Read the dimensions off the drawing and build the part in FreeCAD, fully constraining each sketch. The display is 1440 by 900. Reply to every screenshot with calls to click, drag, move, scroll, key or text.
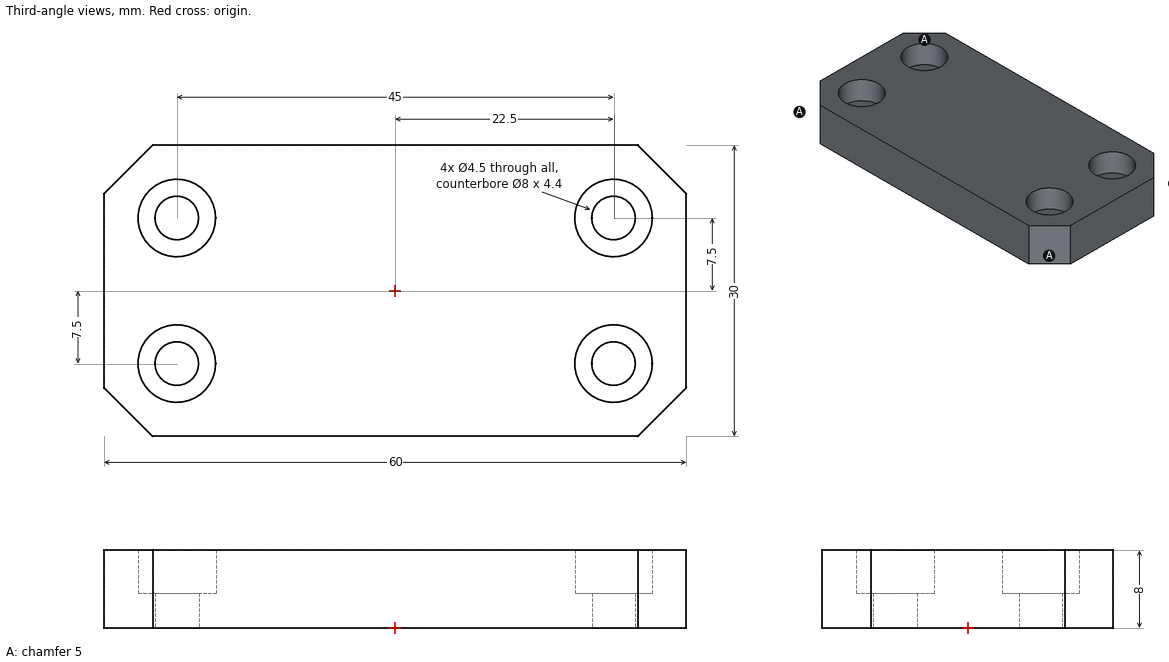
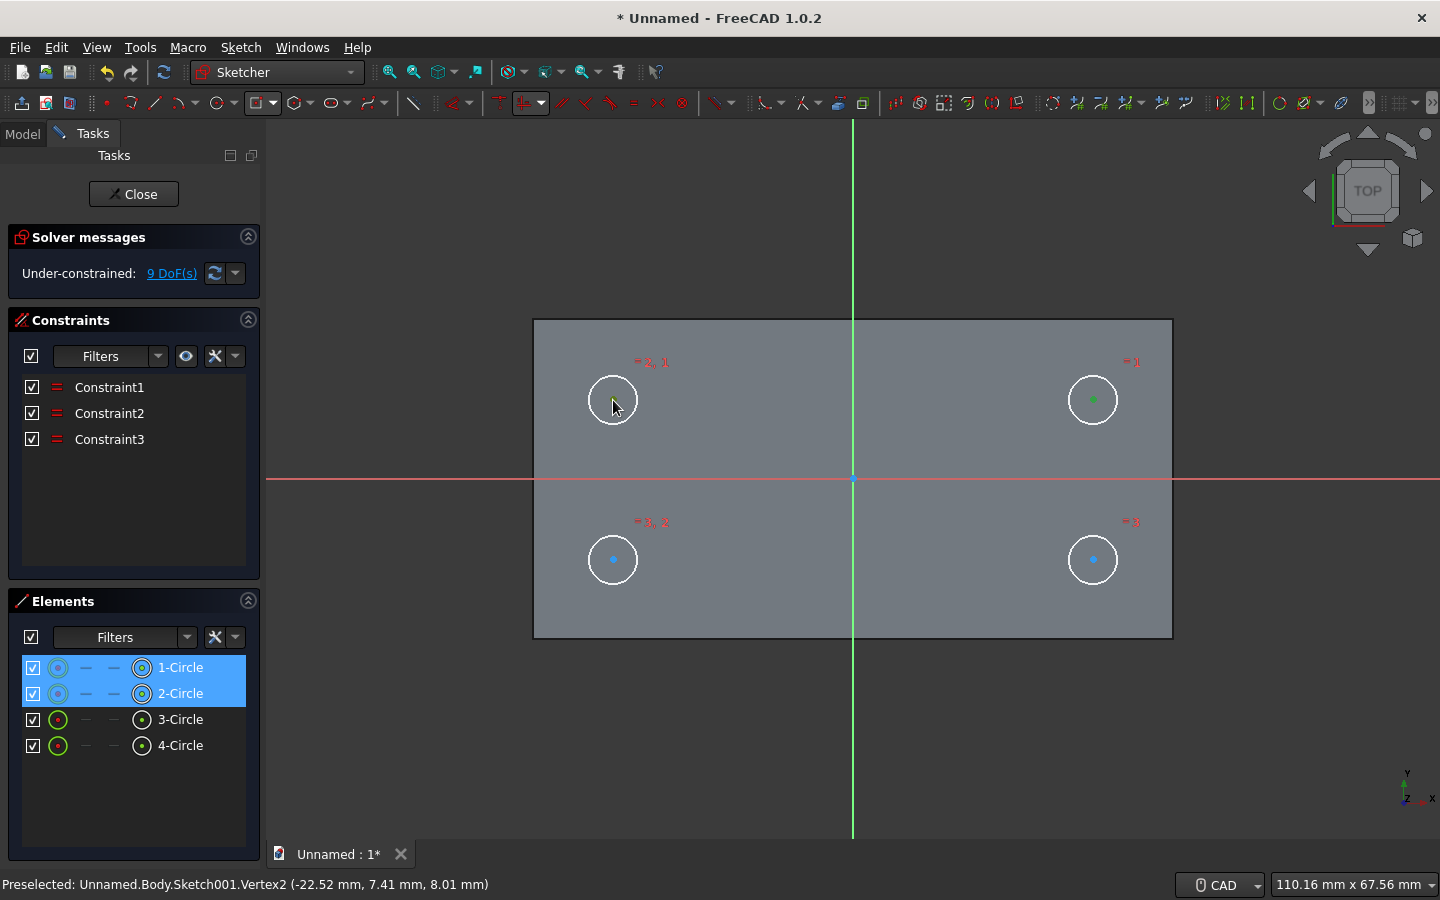
click(544, 104)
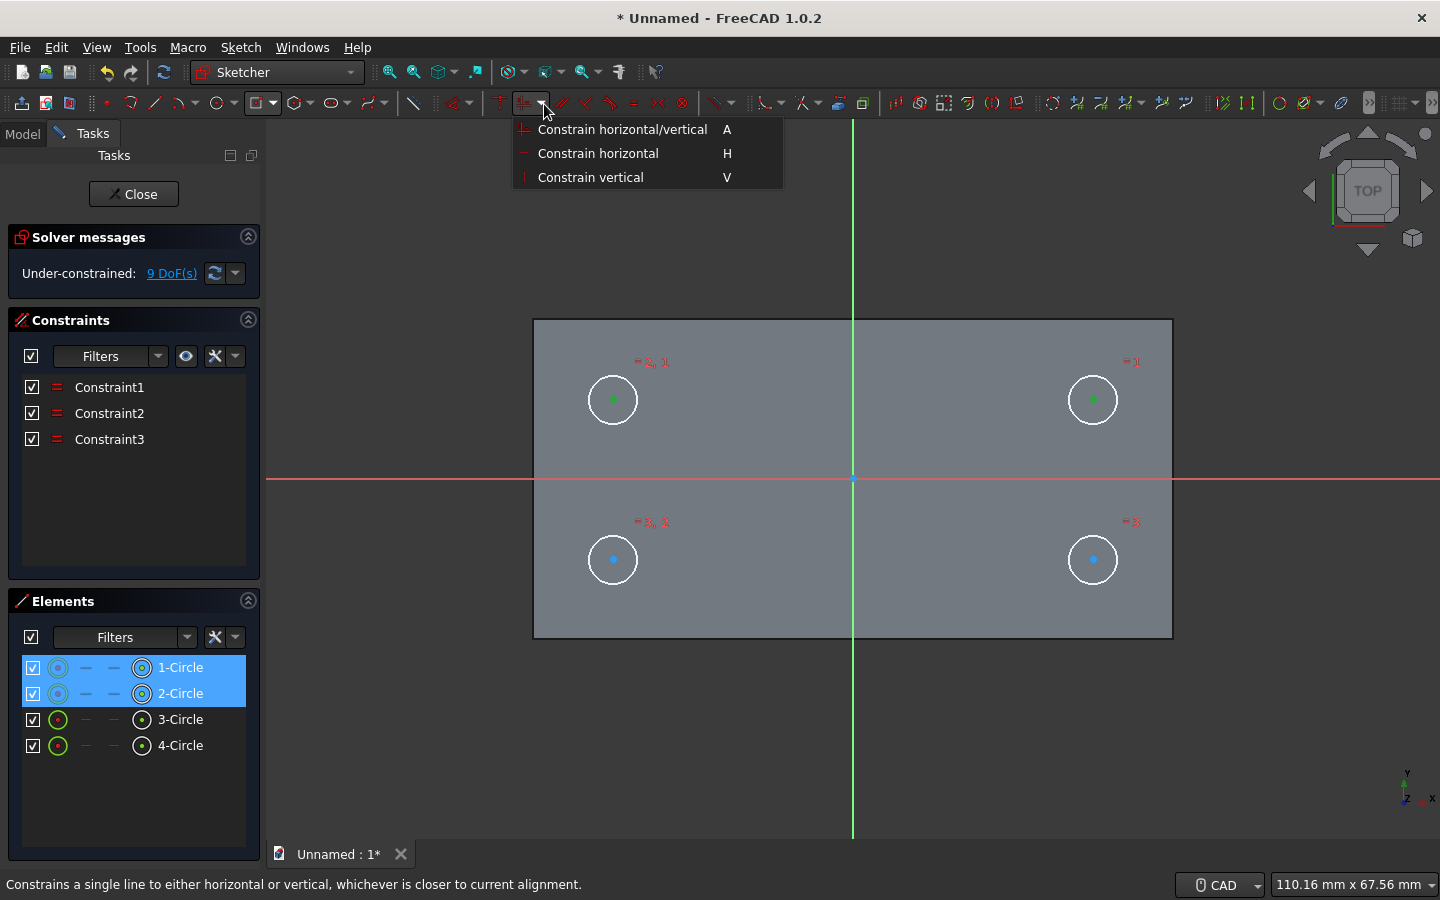
click(648, 153)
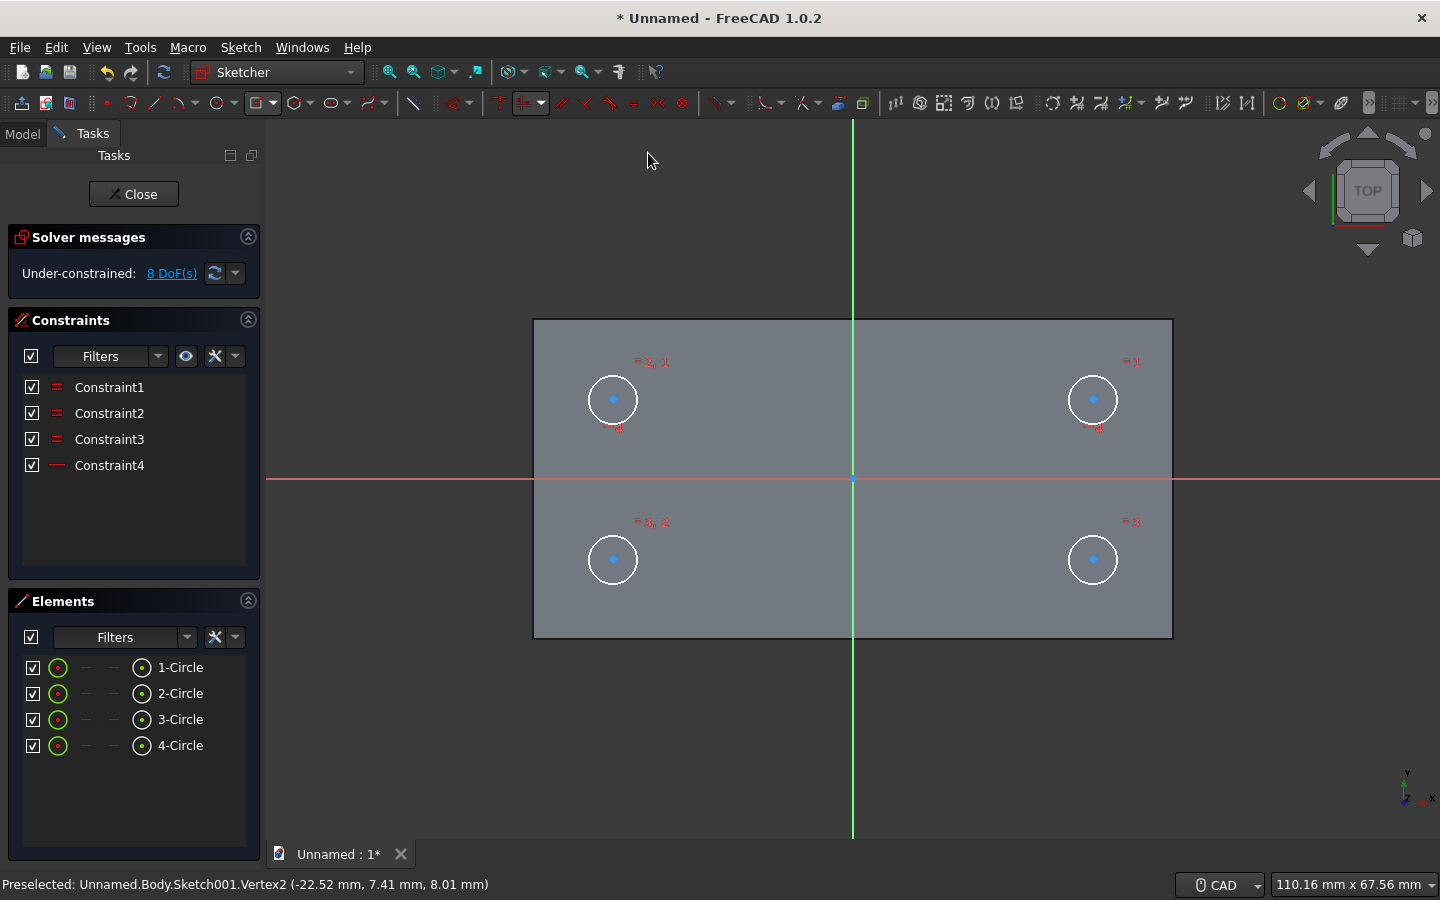
click(613, 400)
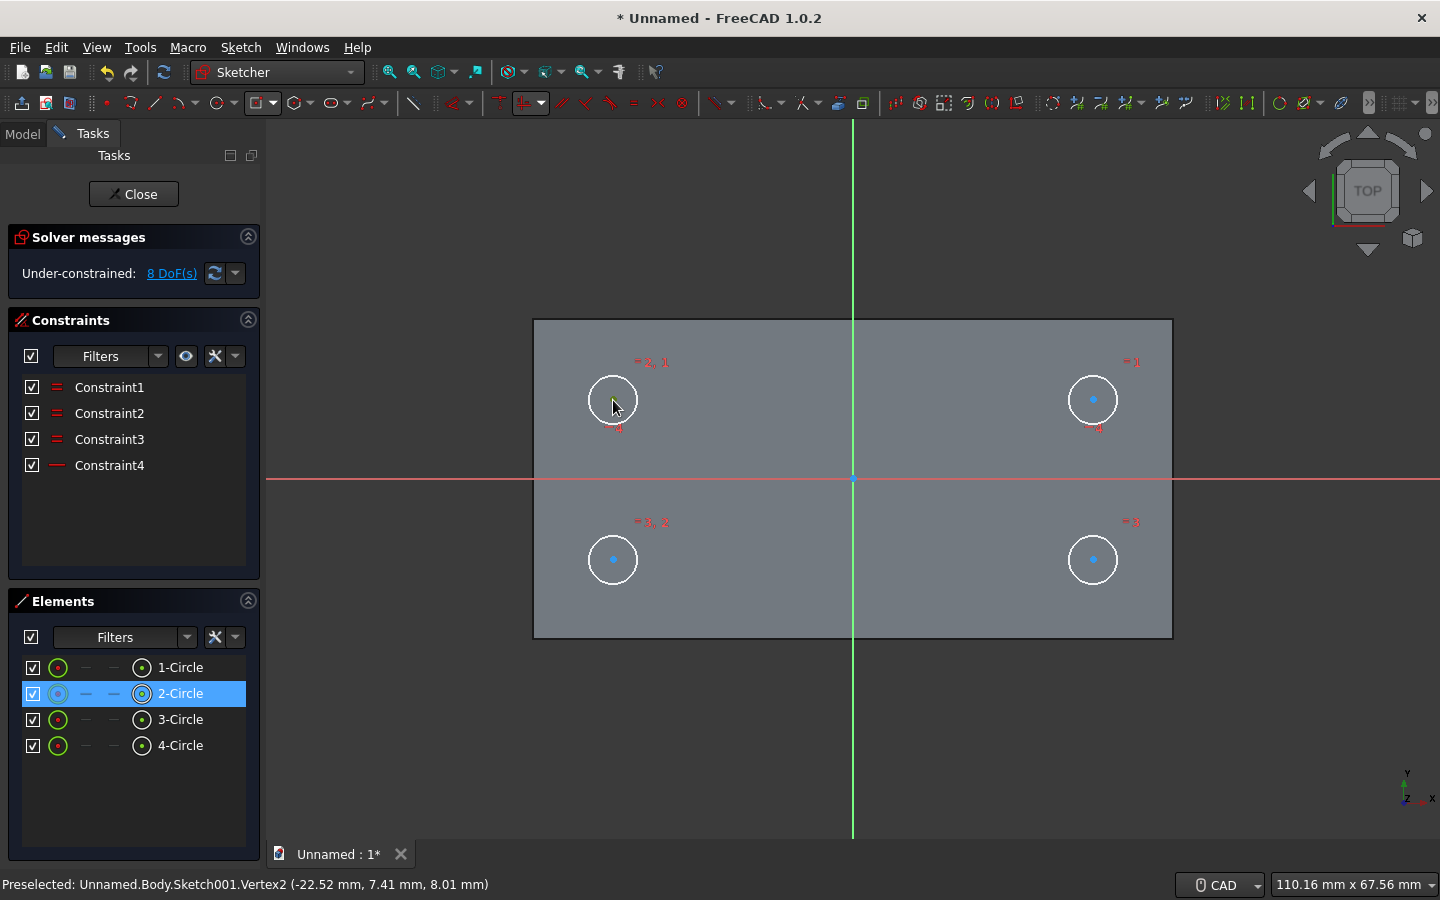
click(613, 560)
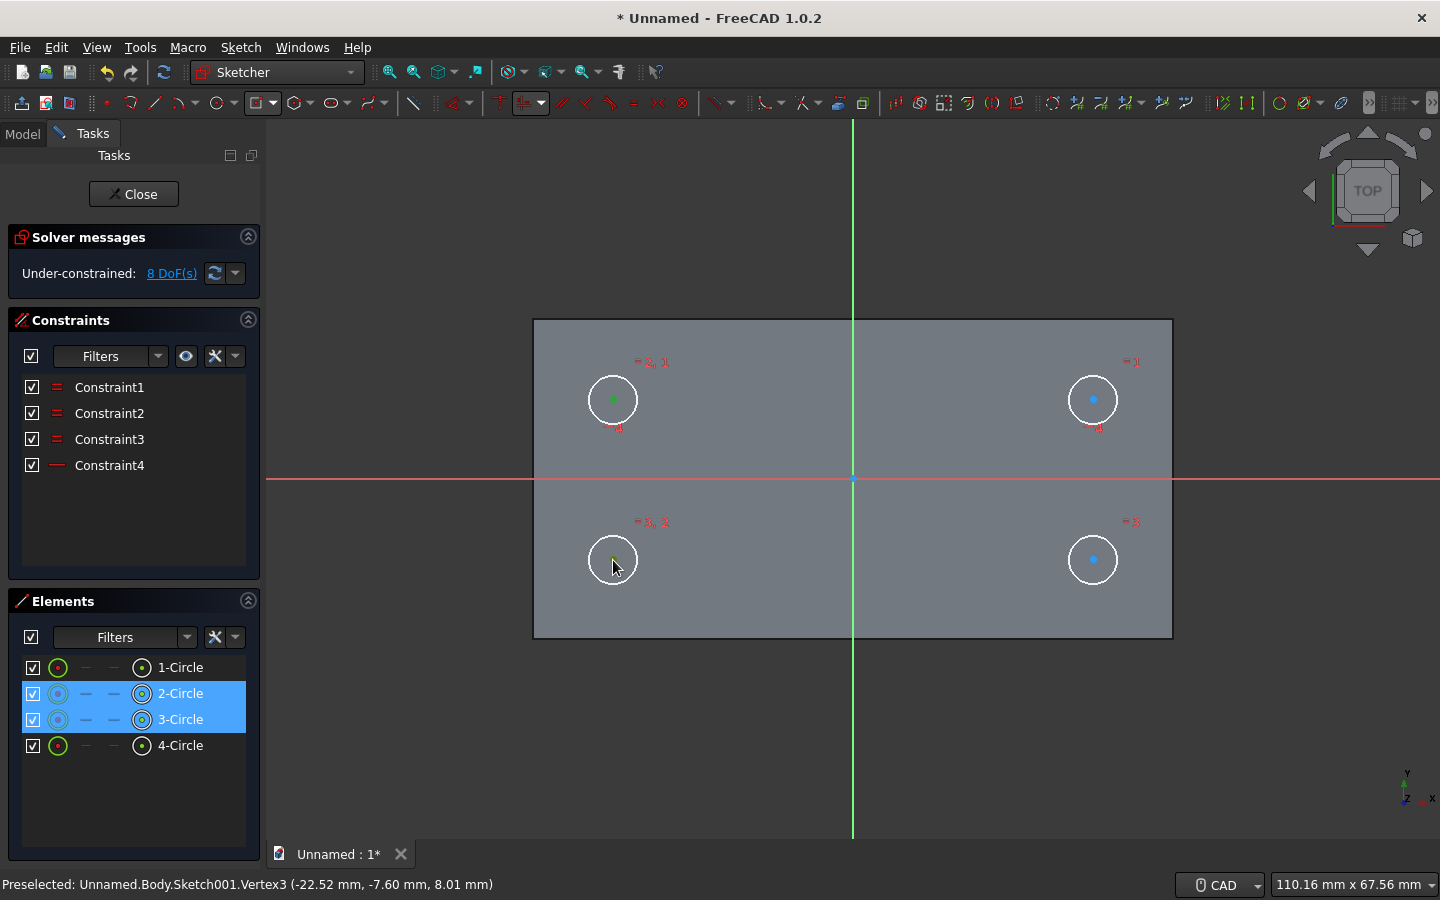
key(v)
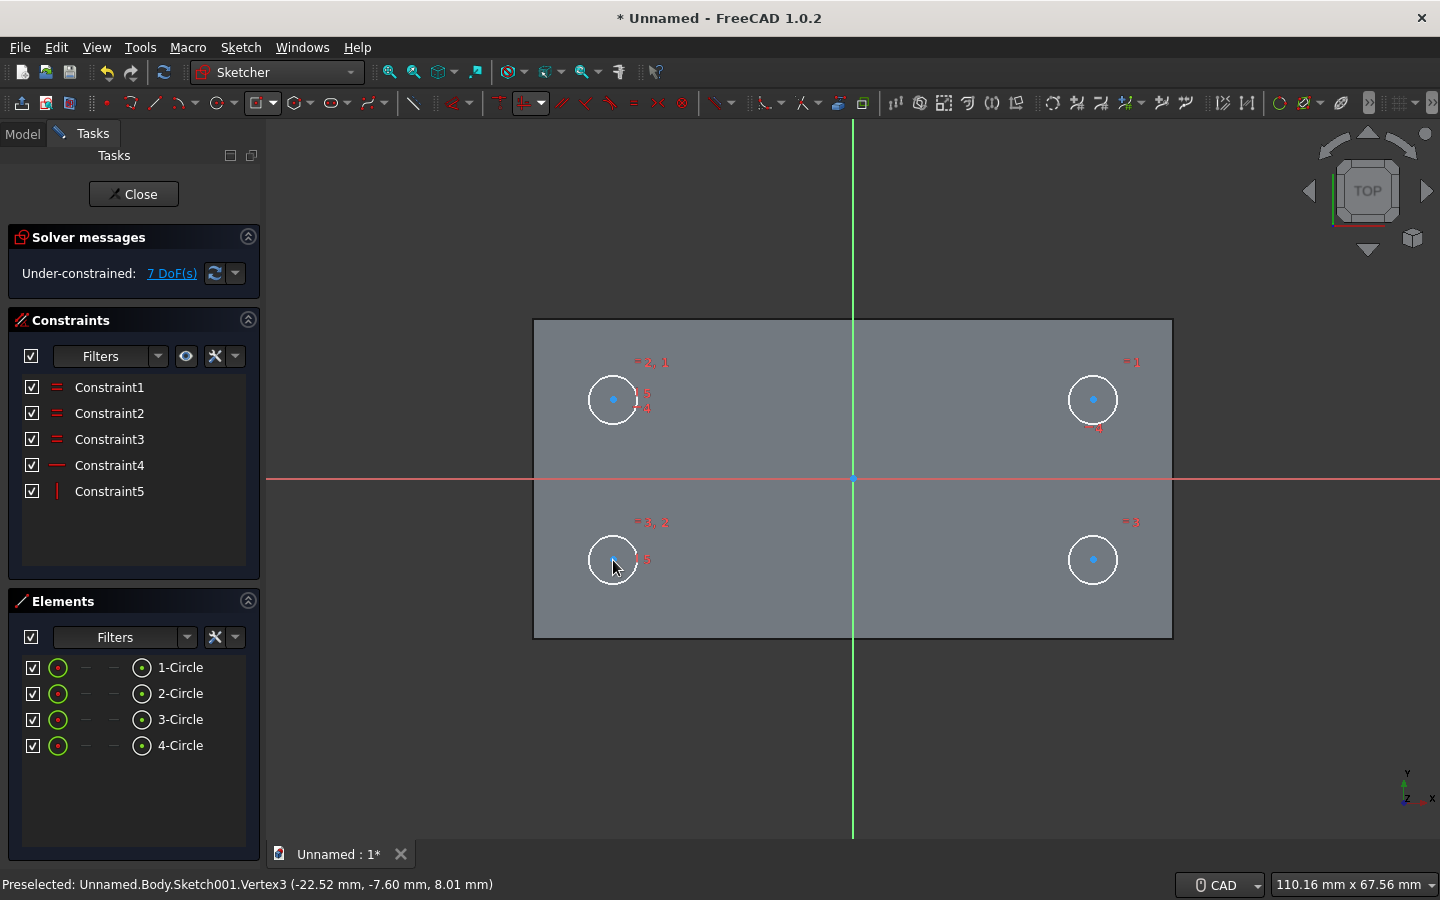
click(1093, 400)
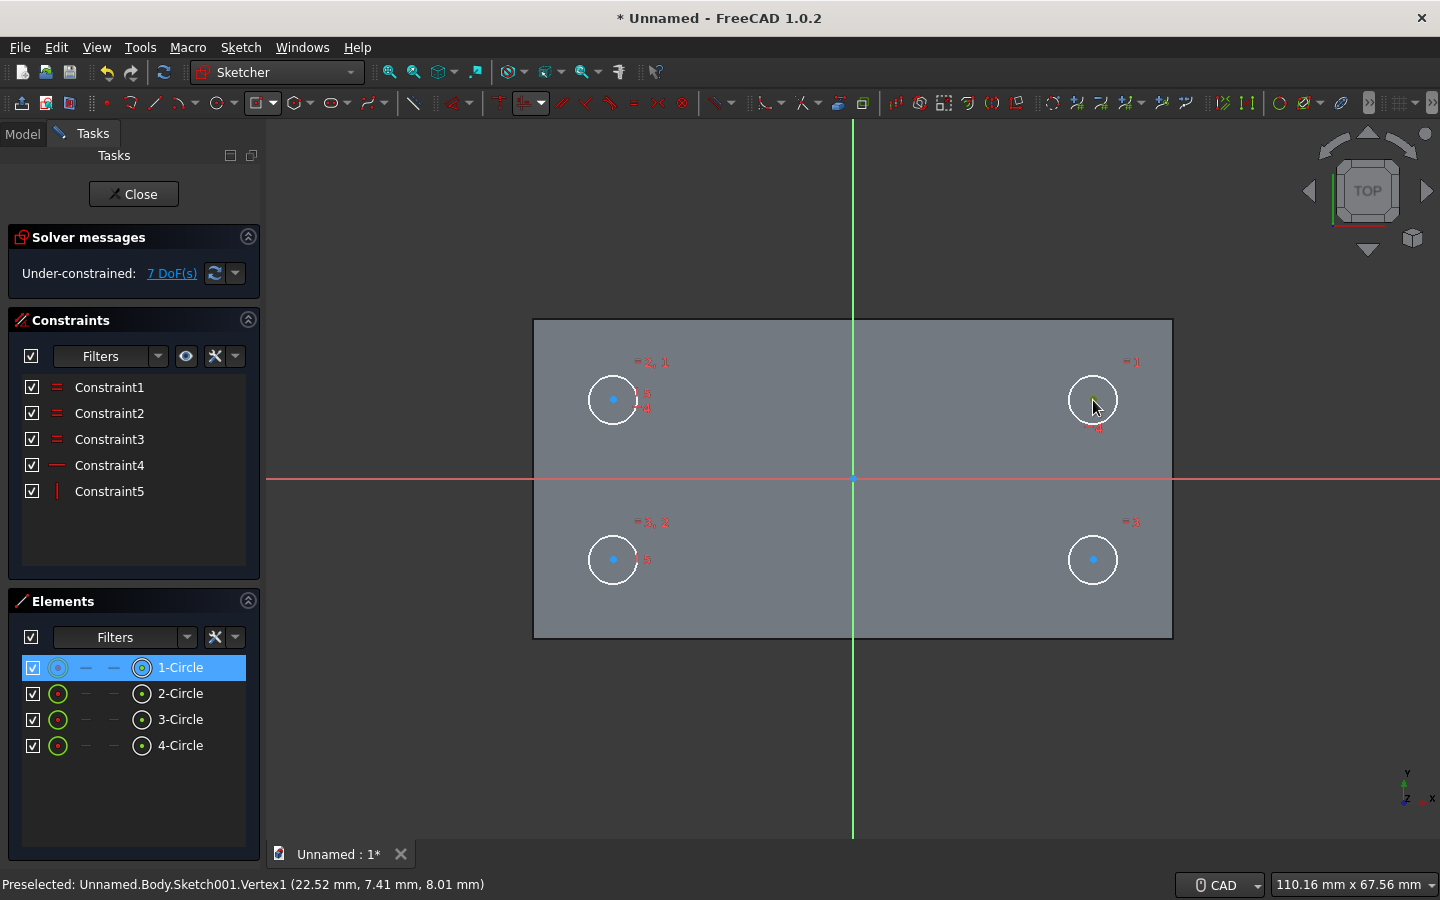
click(1093, 560)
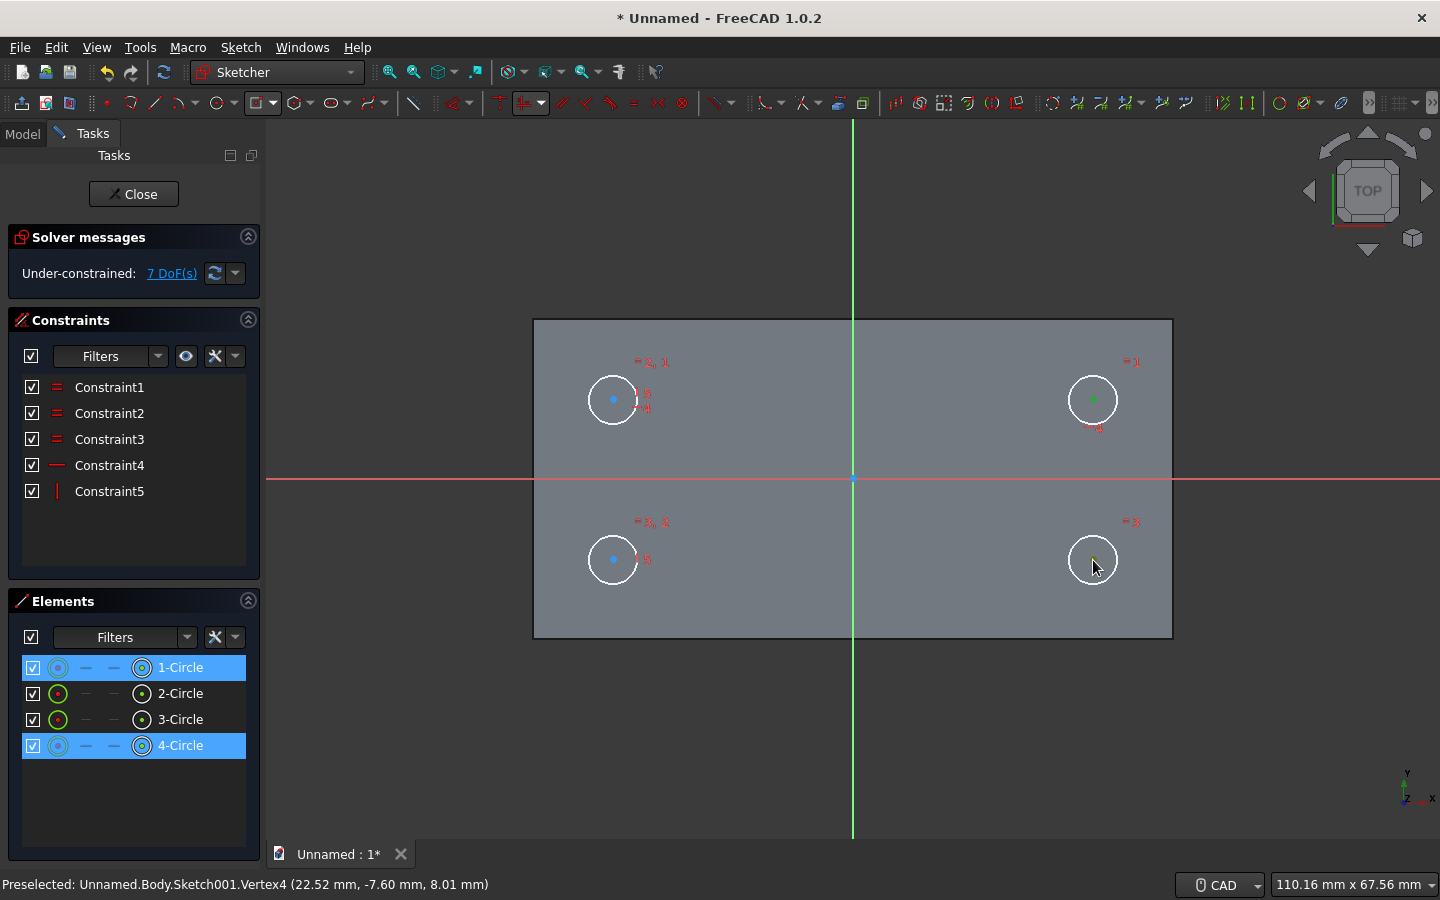
key(v)